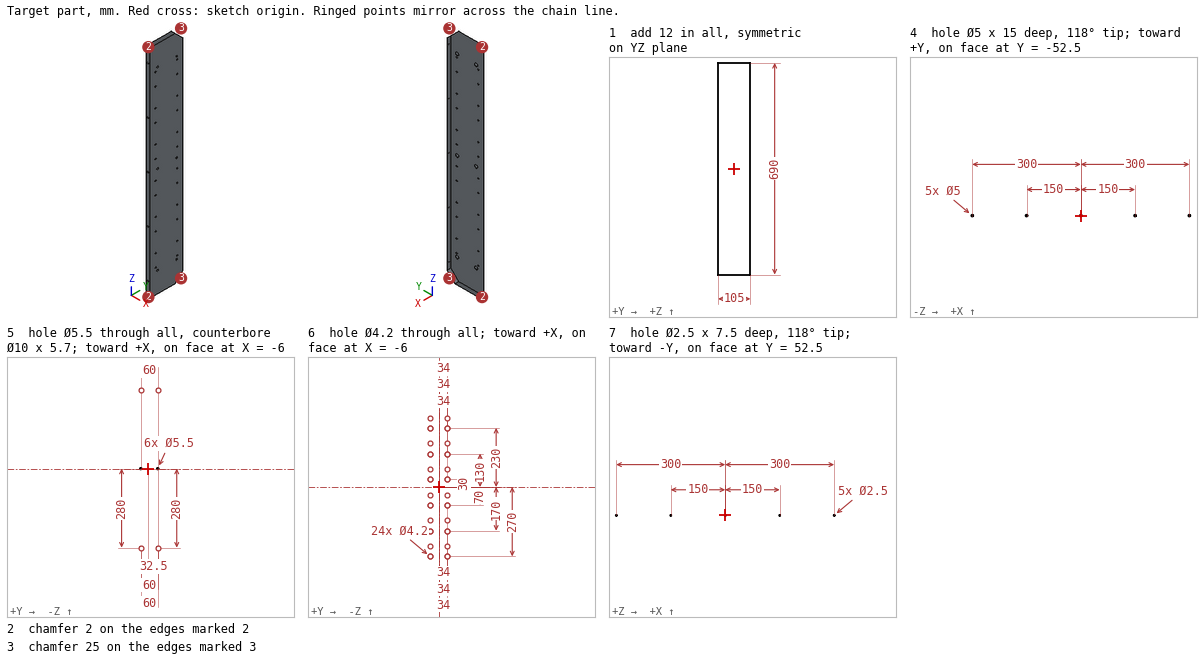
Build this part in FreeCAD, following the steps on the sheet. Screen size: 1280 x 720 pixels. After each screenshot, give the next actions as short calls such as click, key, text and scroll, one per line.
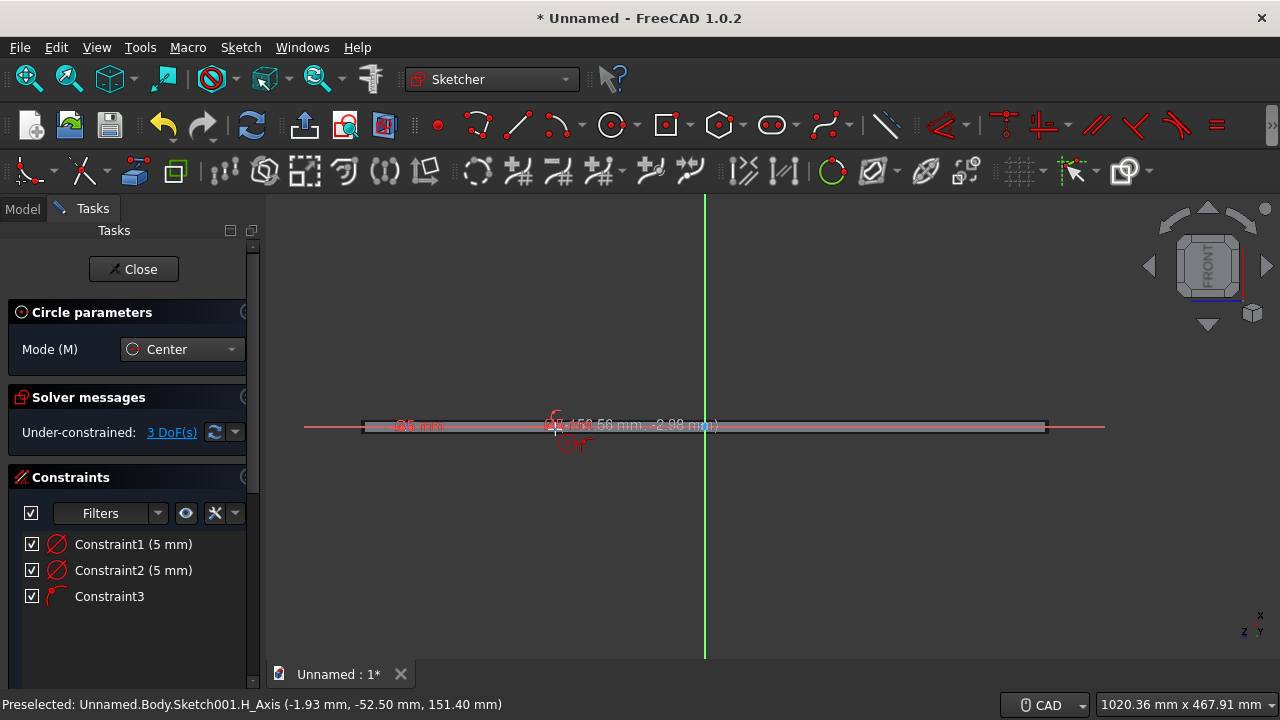
scroll(705, 427, up, 12)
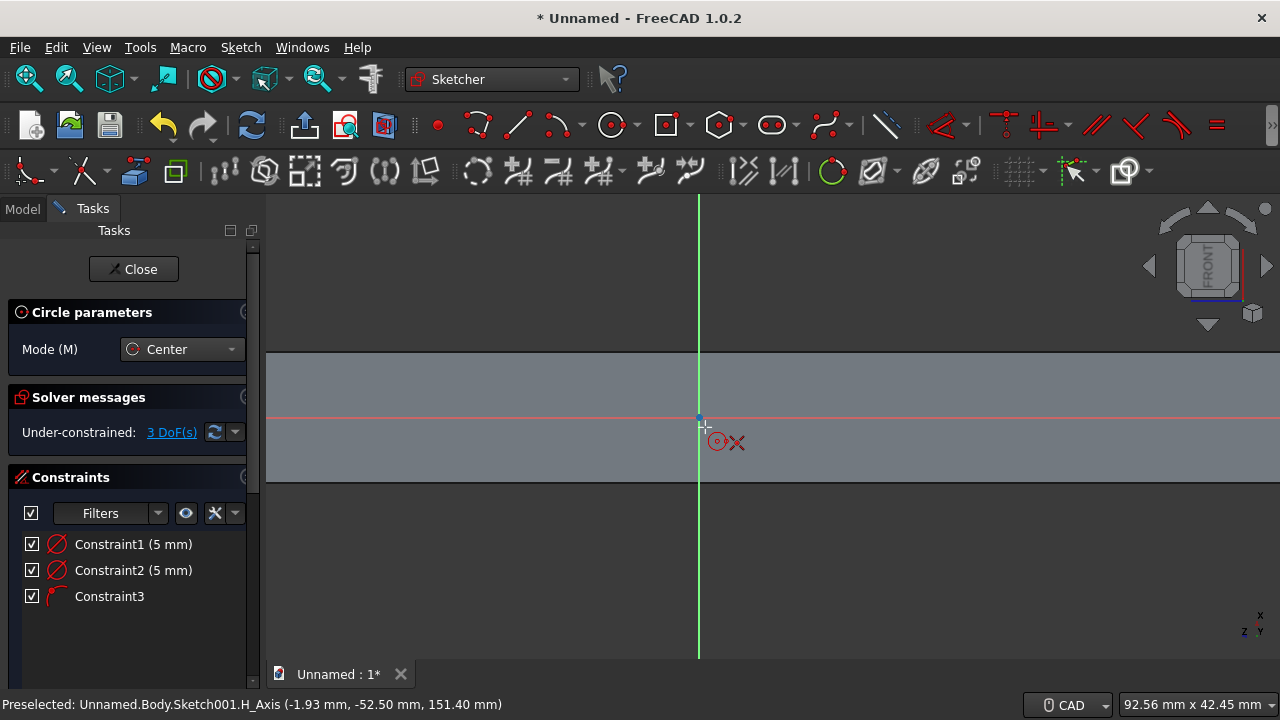
scroll(705, 427, down, 12)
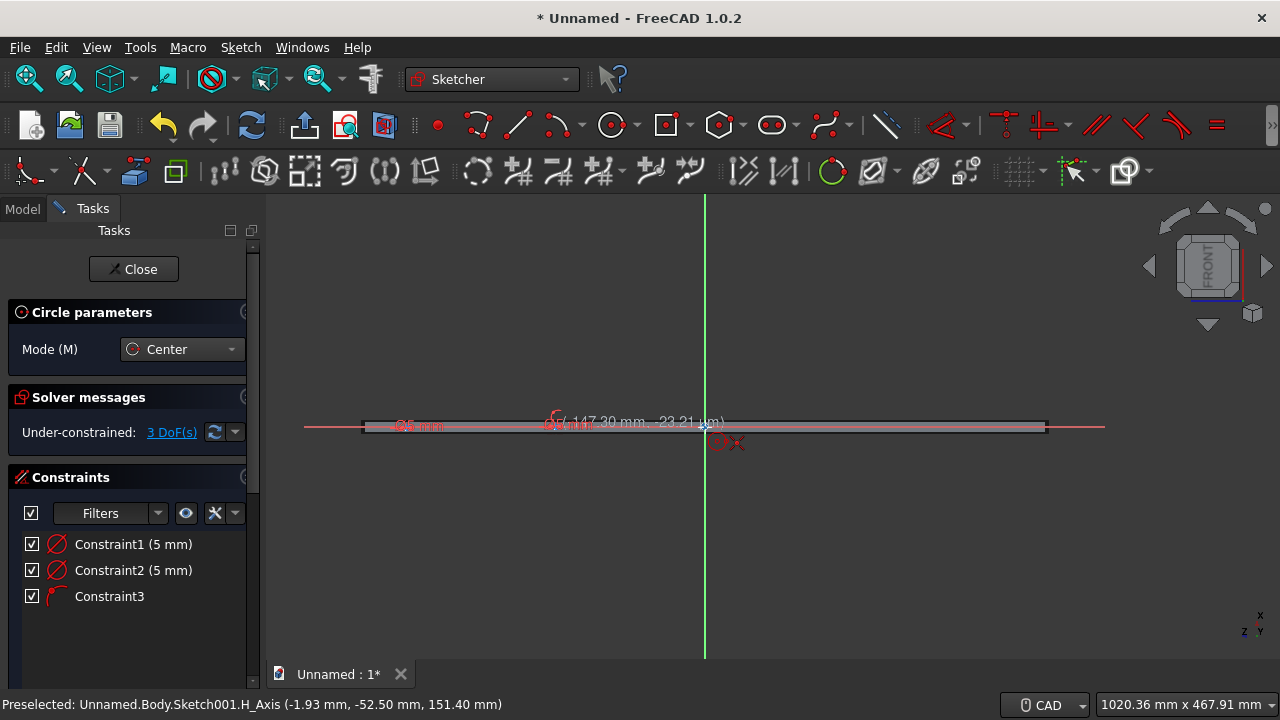
click(705, 427)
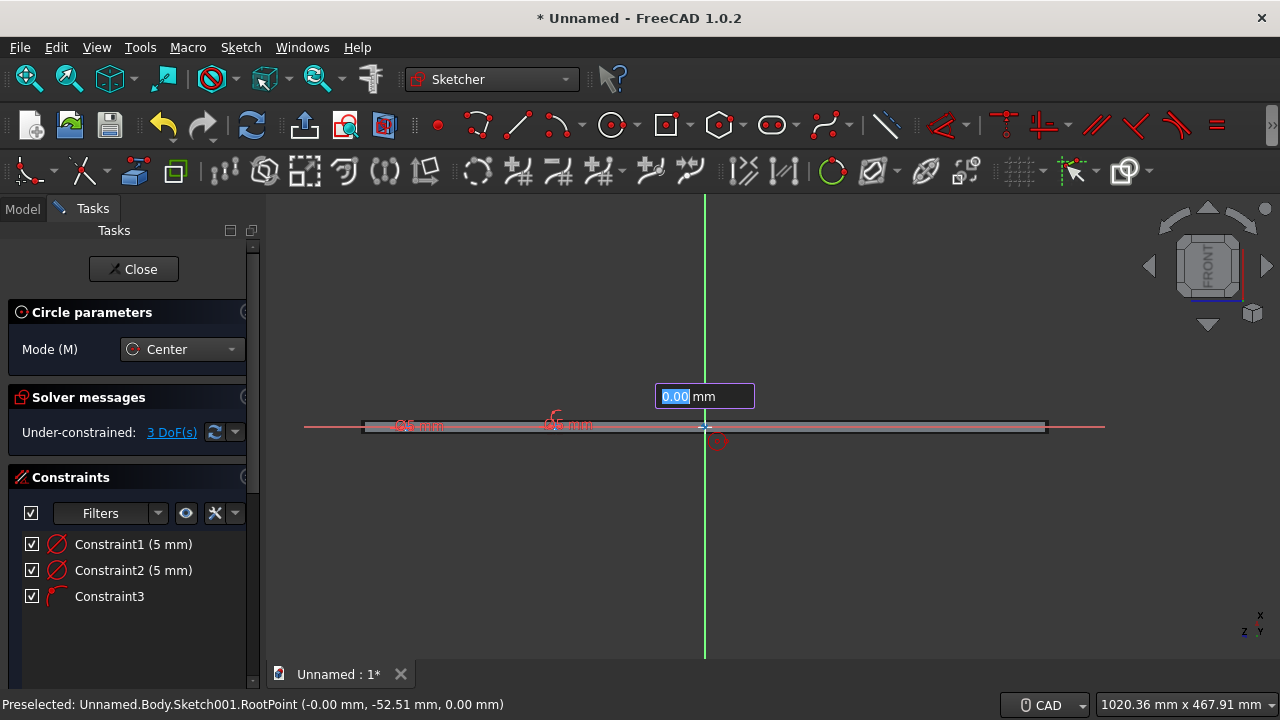
scroll(707, 425, up, 12)
move(699, 418)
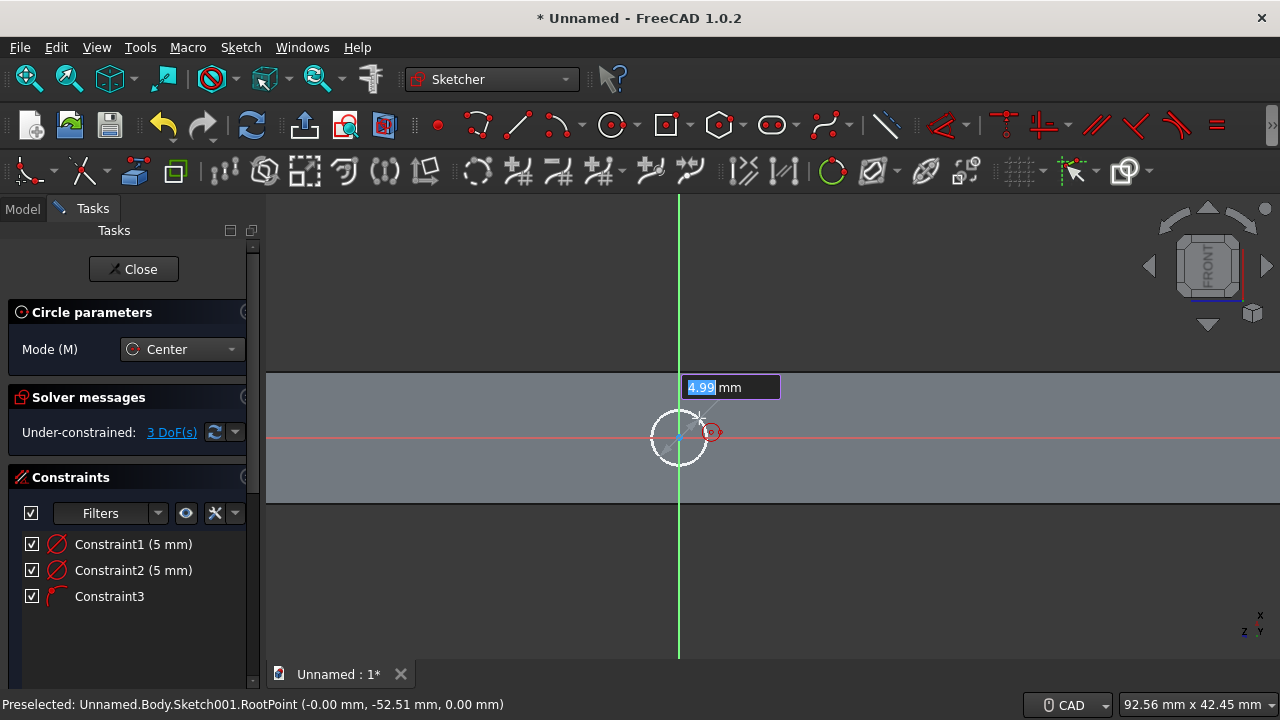
text(5)
key(Return)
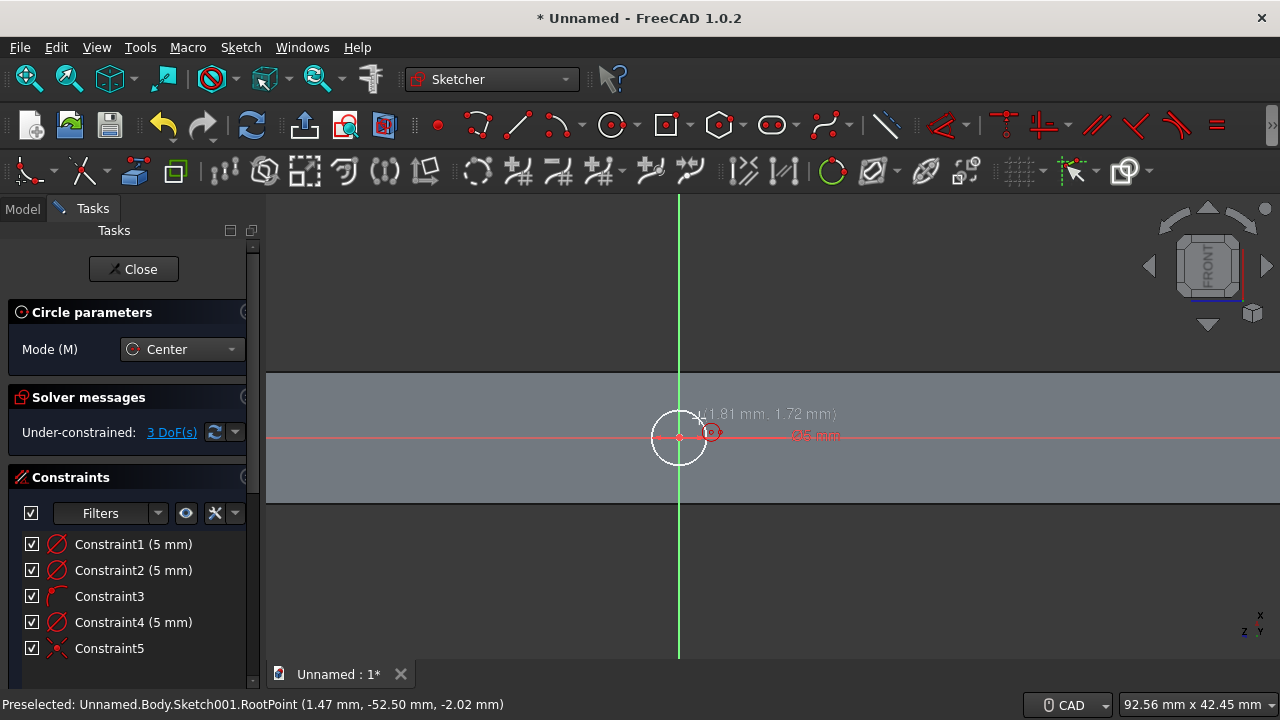
scroll(707, 425, down, 12)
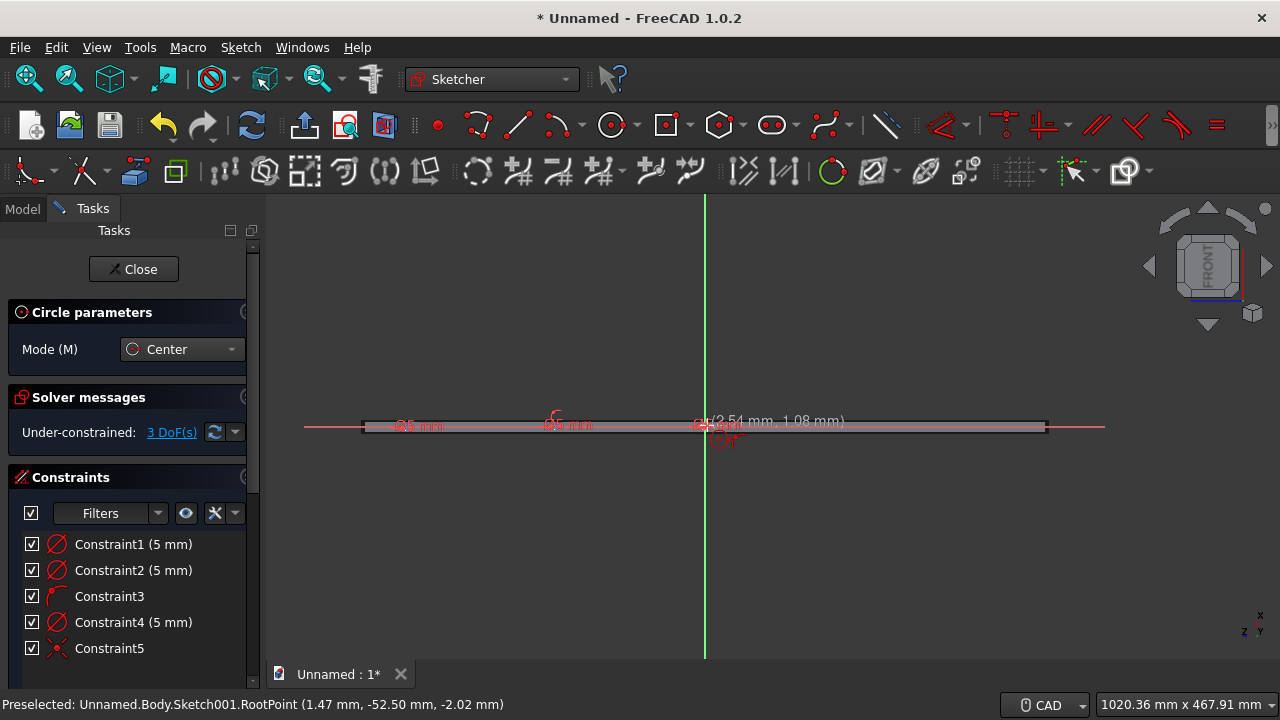
scroll(854, 427, up, 12)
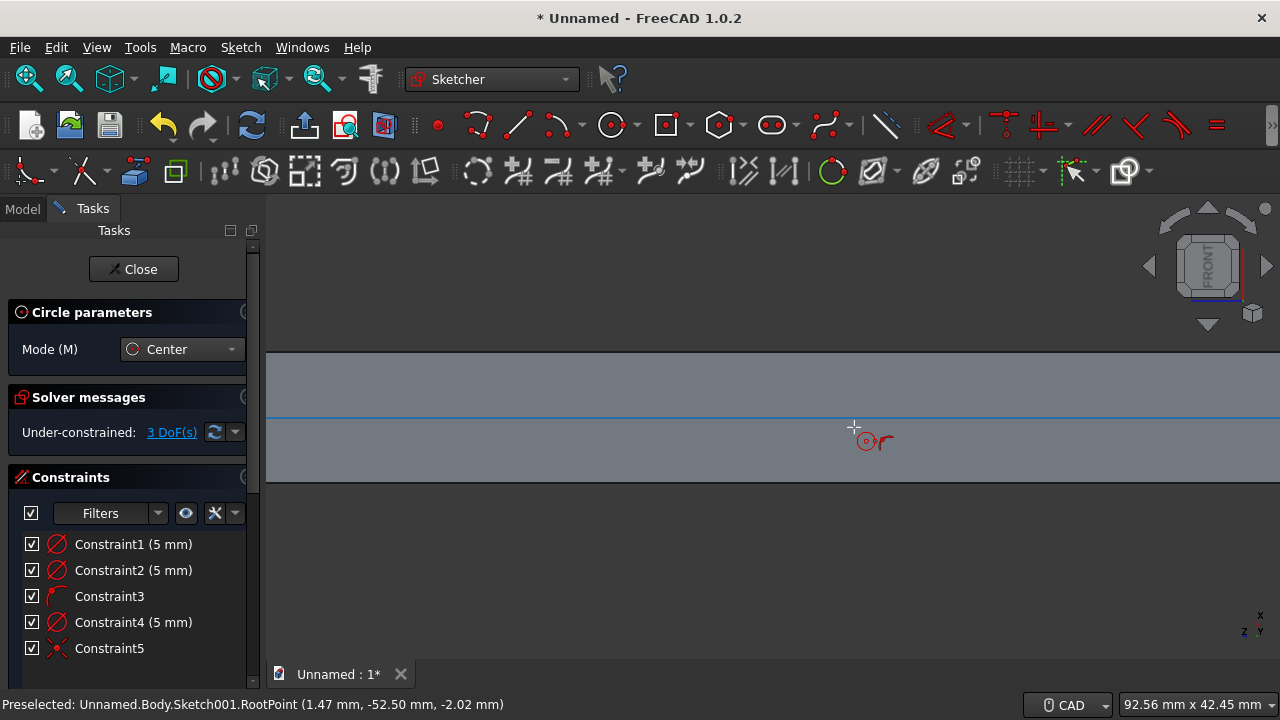
scroll(854, 427, down, 12)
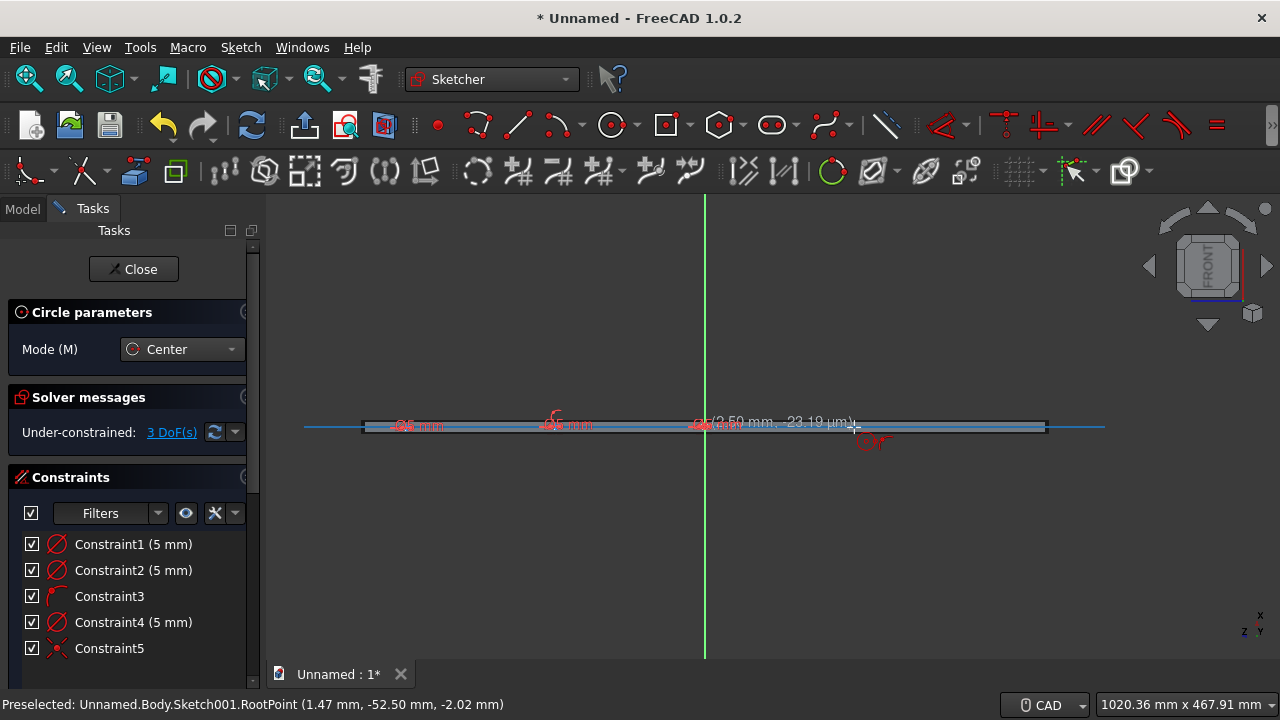
click(854, 427)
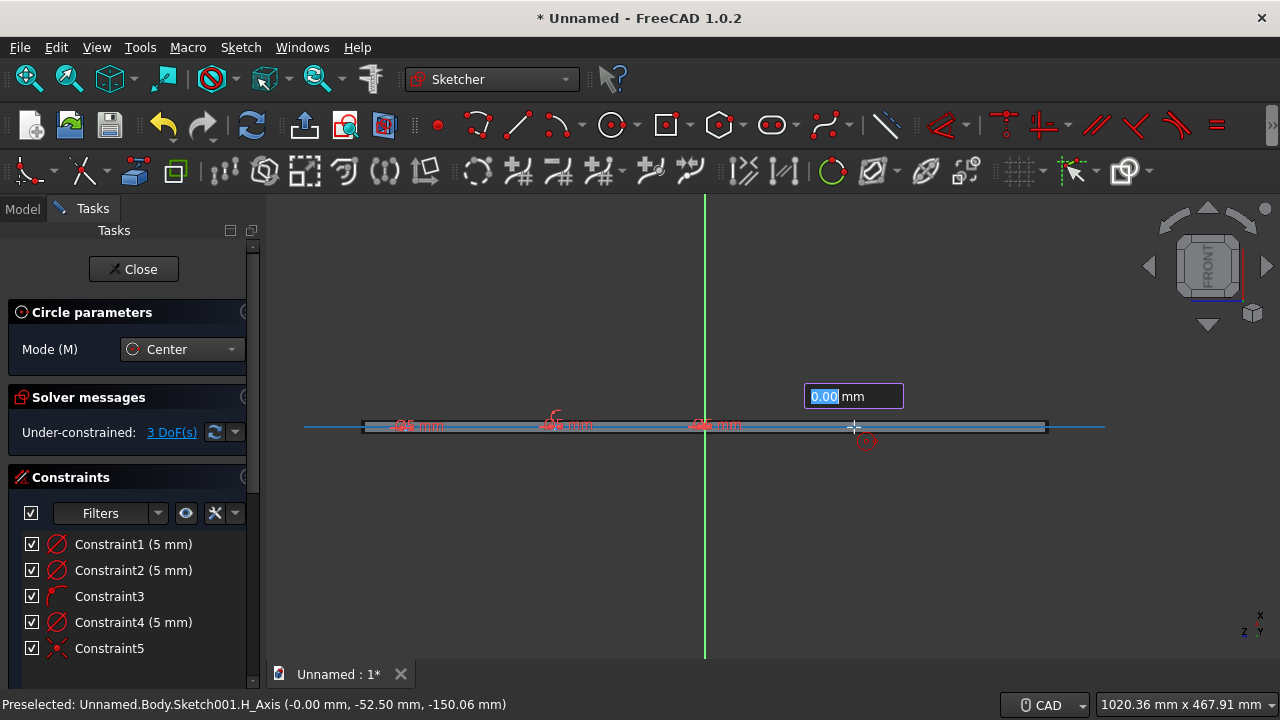
scroll(853, 429, up, 10)
move(850, 425)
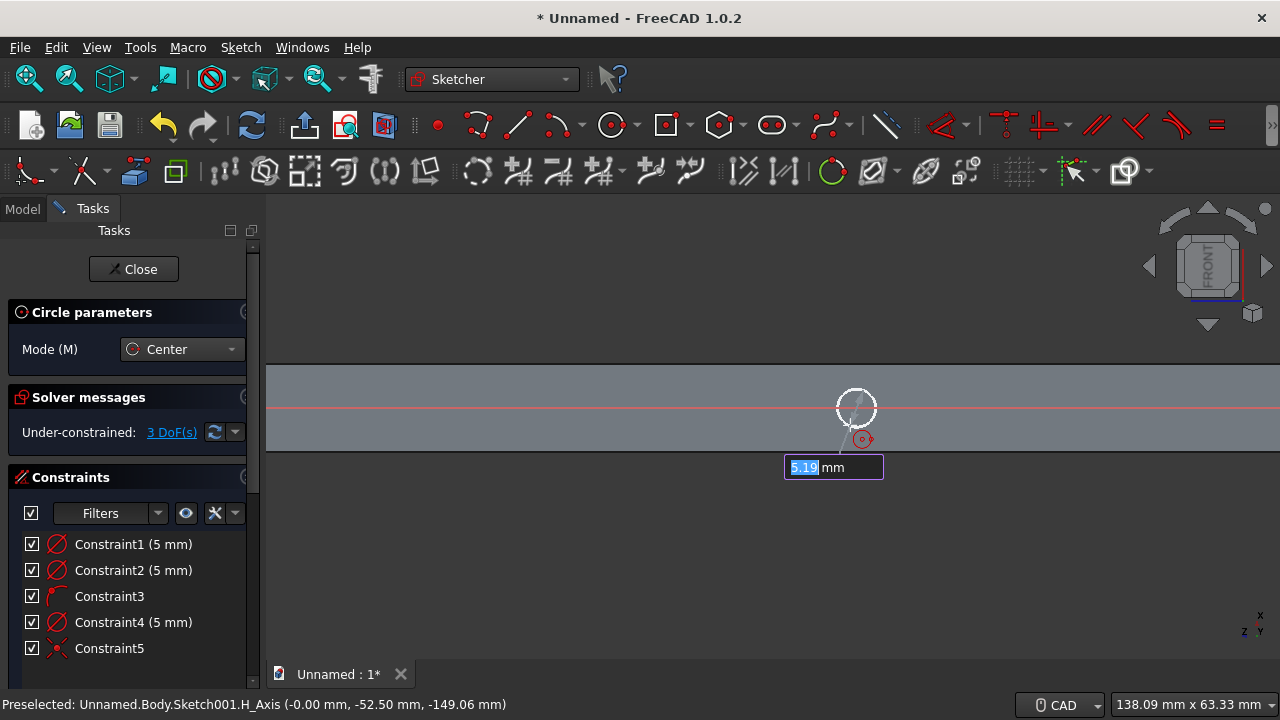
text(5)
key(Return)